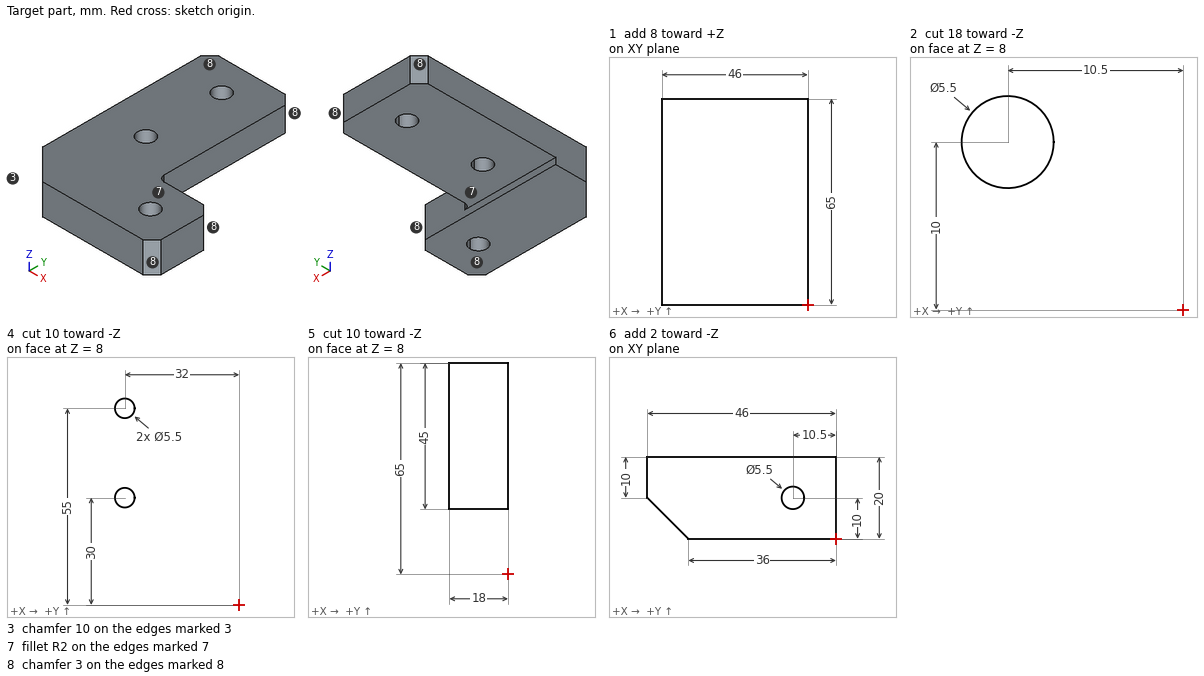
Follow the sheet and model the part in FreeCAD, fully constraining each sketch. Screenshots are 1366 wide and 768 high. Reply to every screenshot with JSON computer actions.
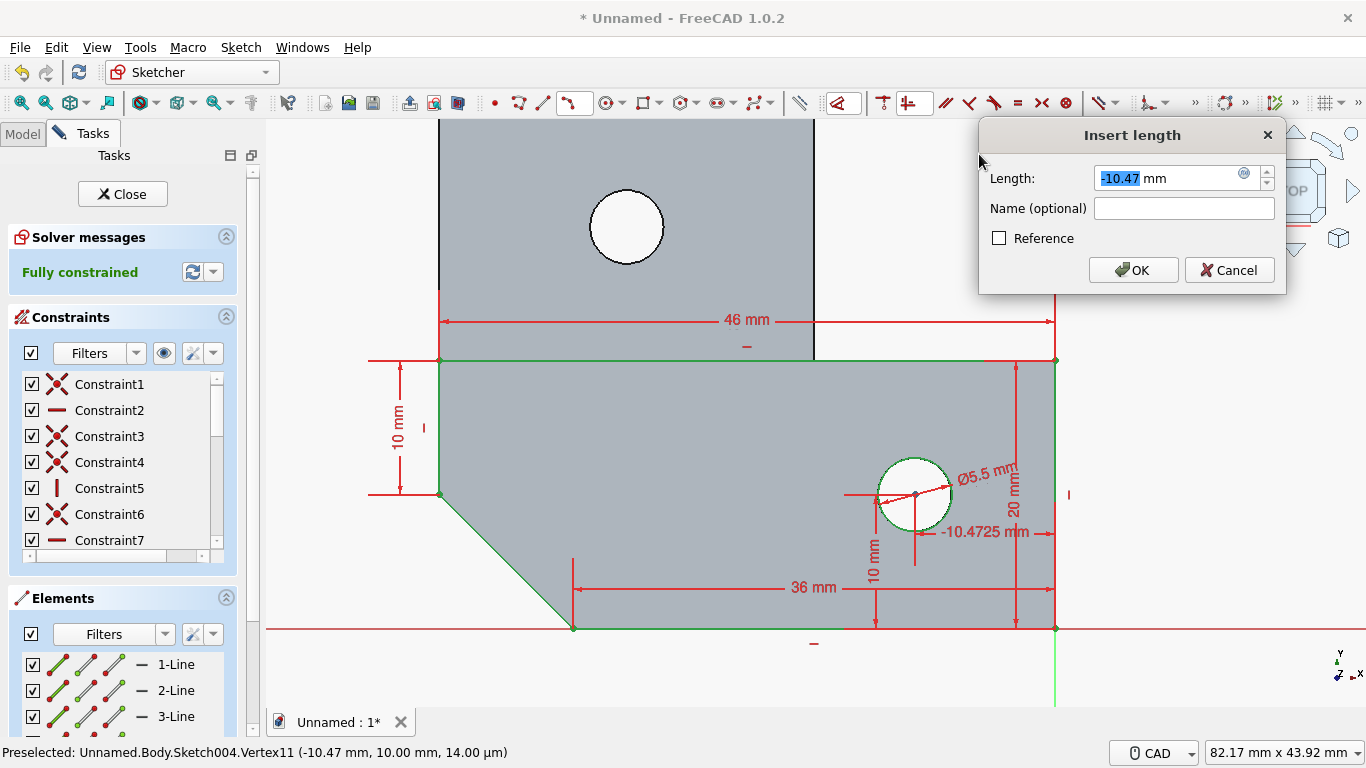
{"action": "type", "text": "-10.5"}
{"action": "key", "text": "Return"}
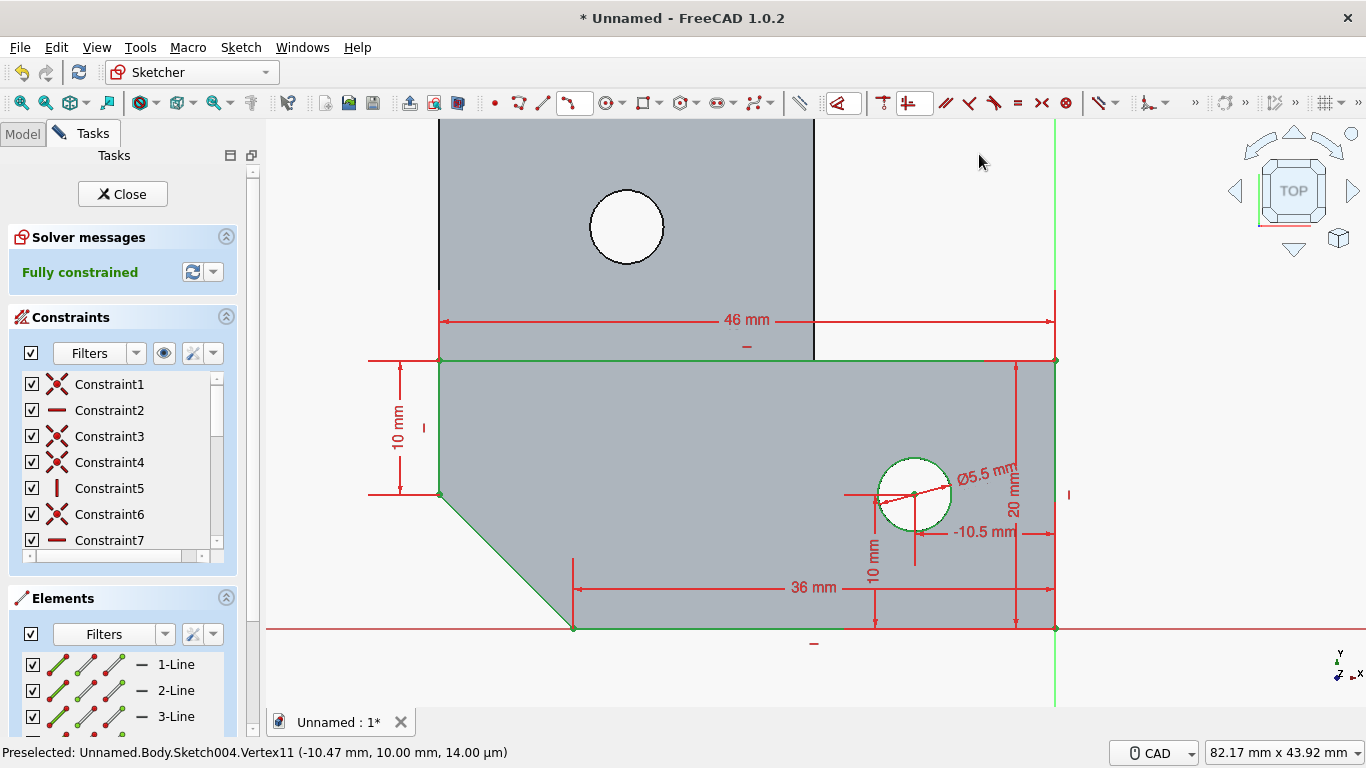
{"action": "left_click", "coordinate": [123, 194]}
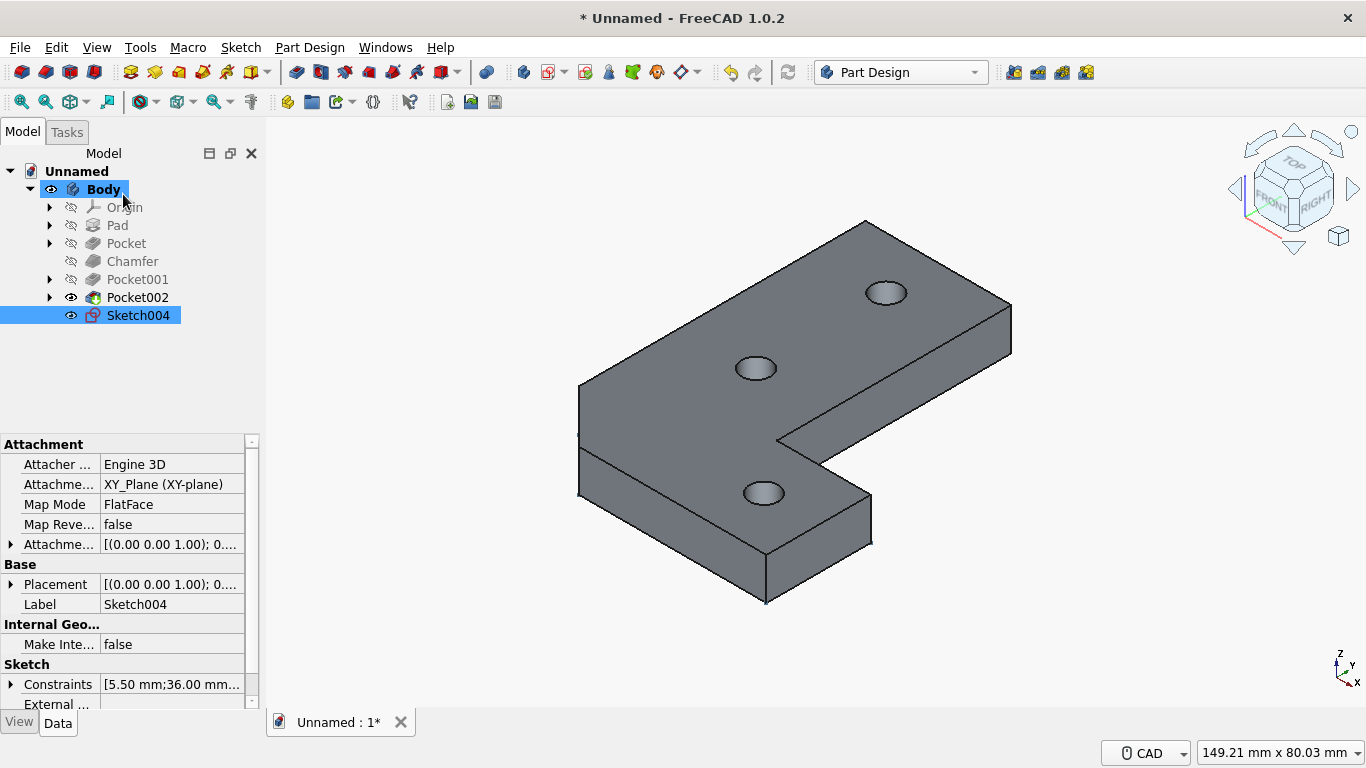
{"action": "left_click", "coordinate": [132, 72]}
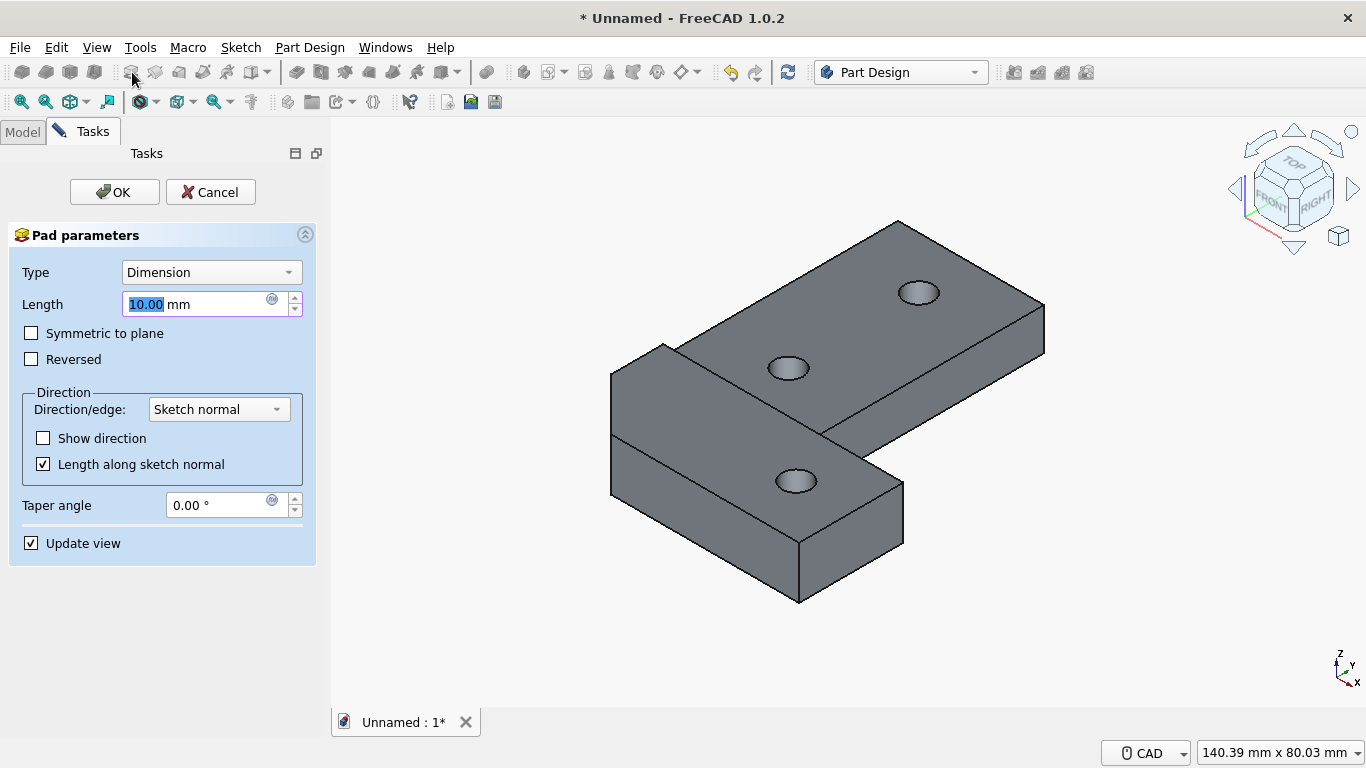
{"action": "type", "text": "2"}
{"action": "key", "text": "Tab"}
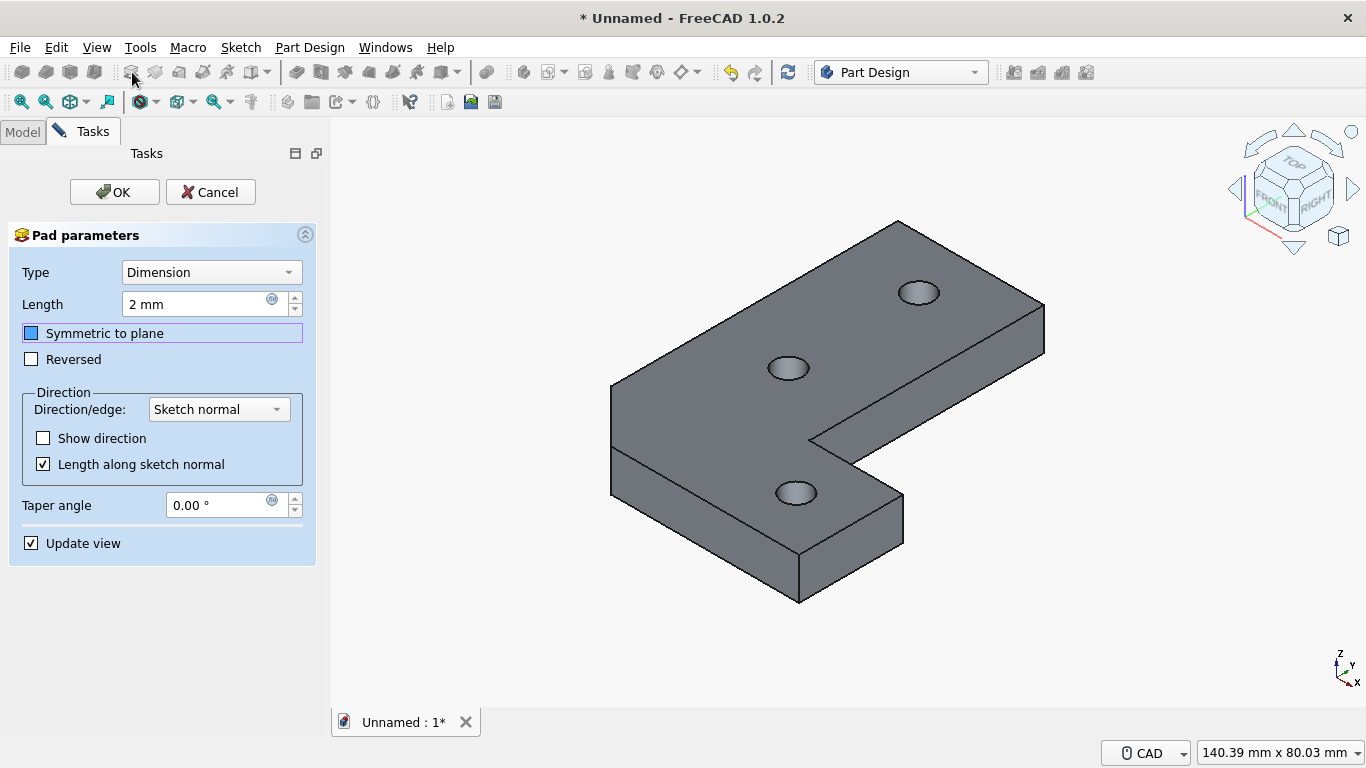
{"action": "left_click", "coordinate": [30, 359]}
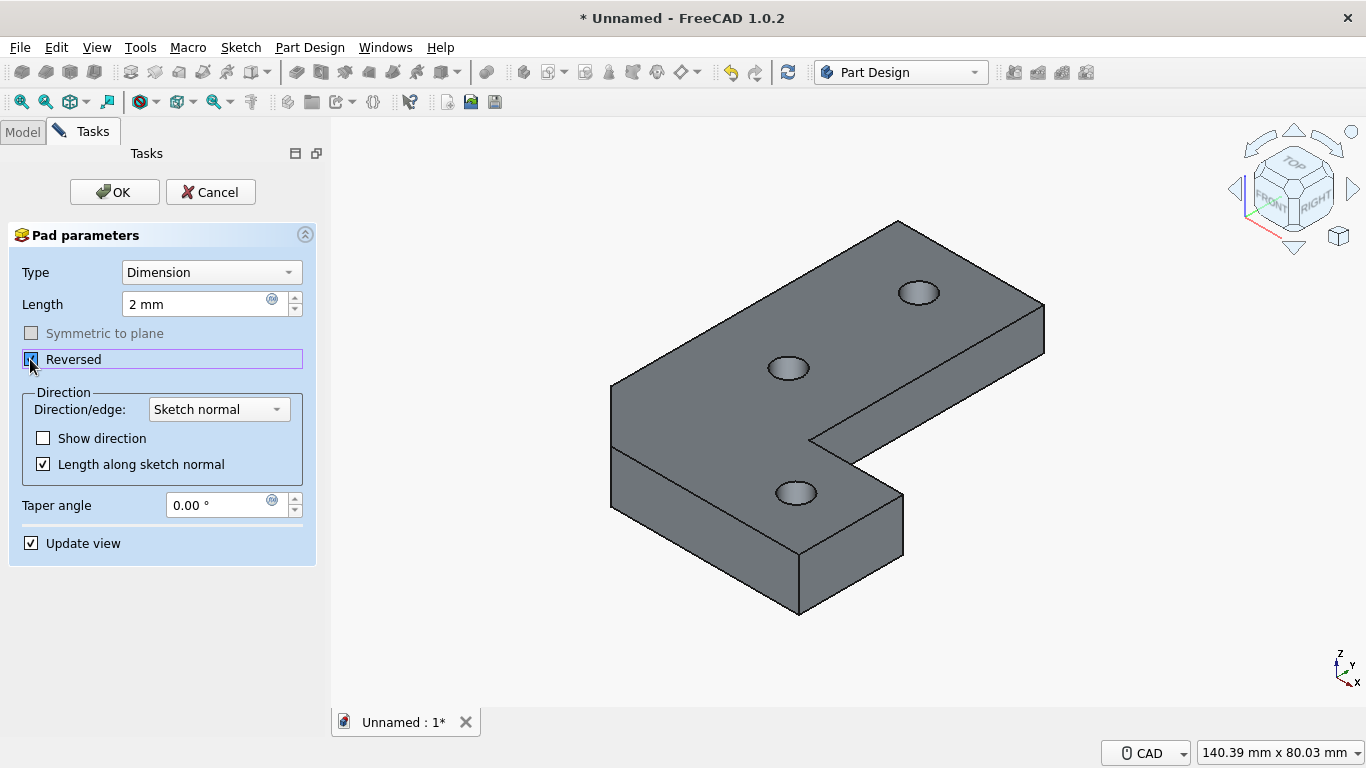
{"action": "left_click", "coordinate": [115, 192]}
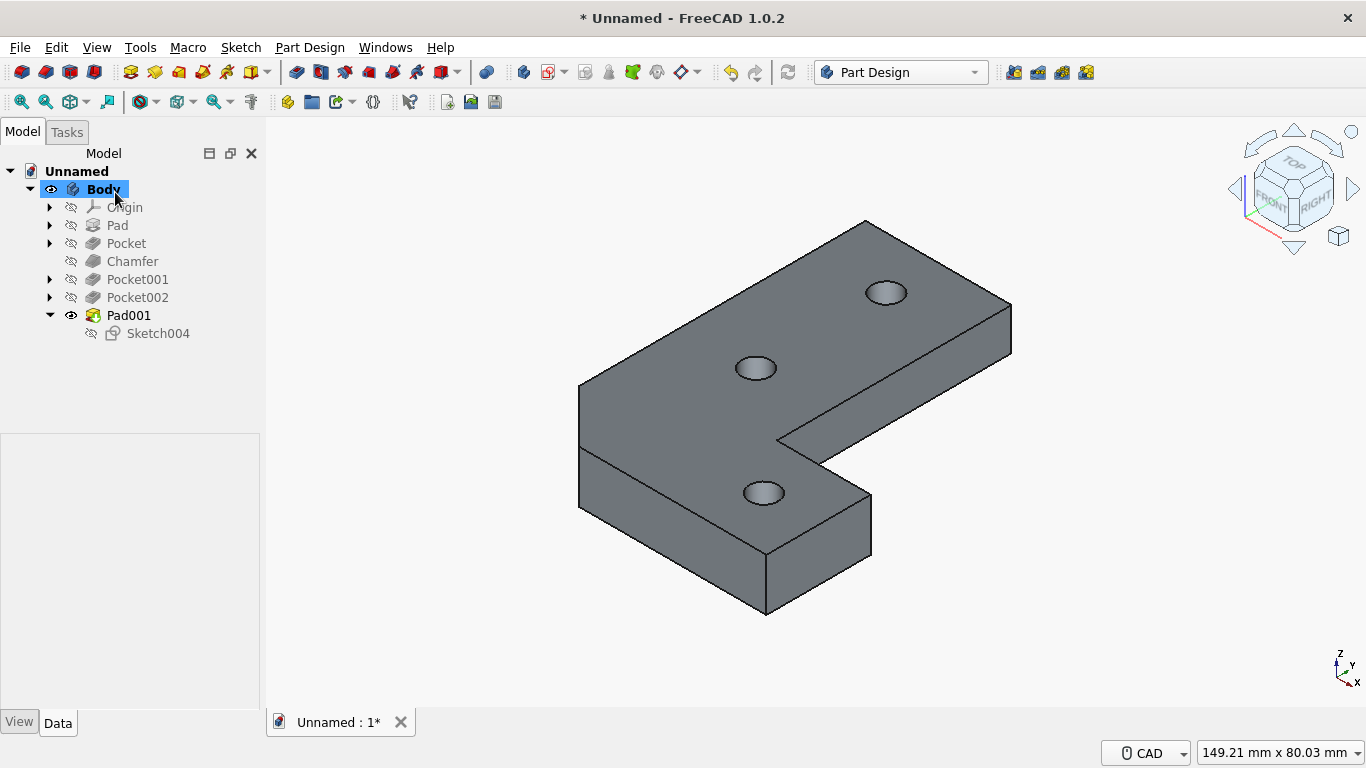
{"action": "key", "text": "2"}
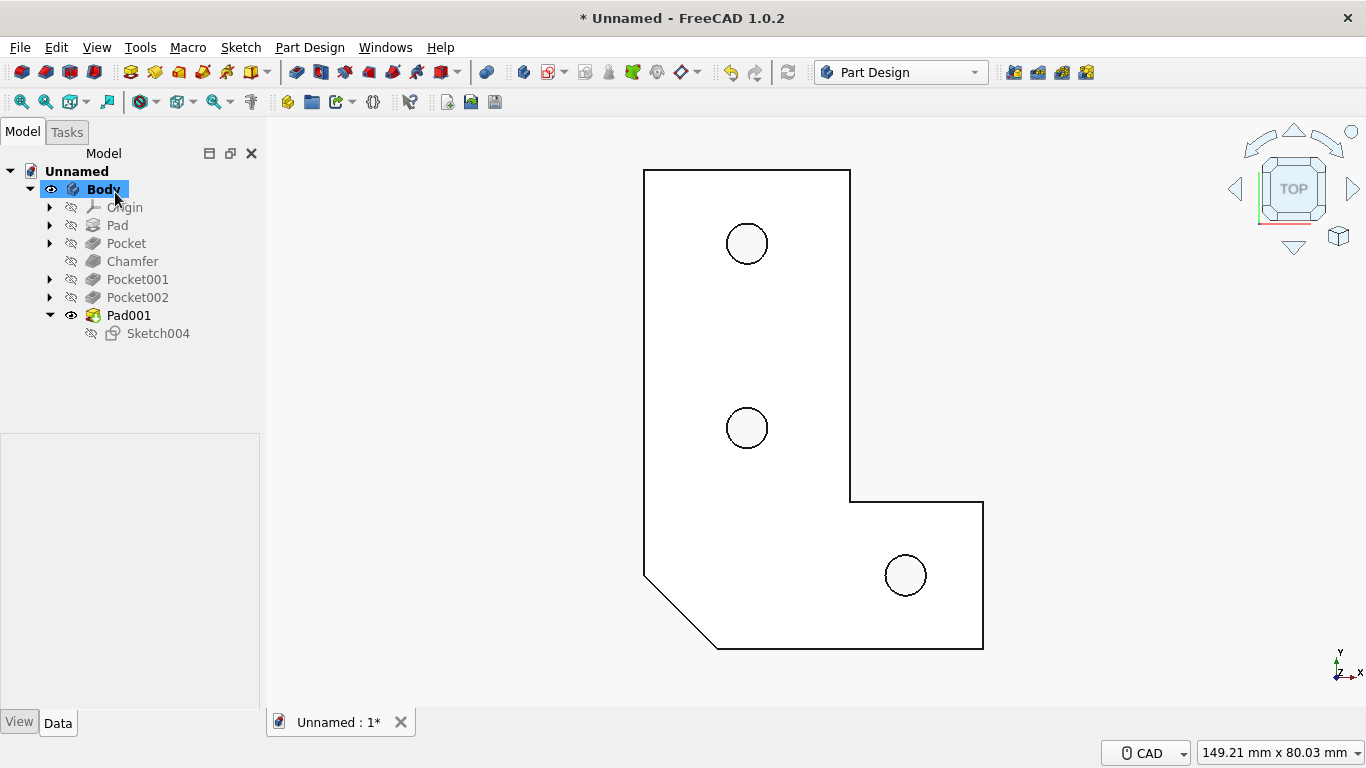
{"action": "key", "text": "0"}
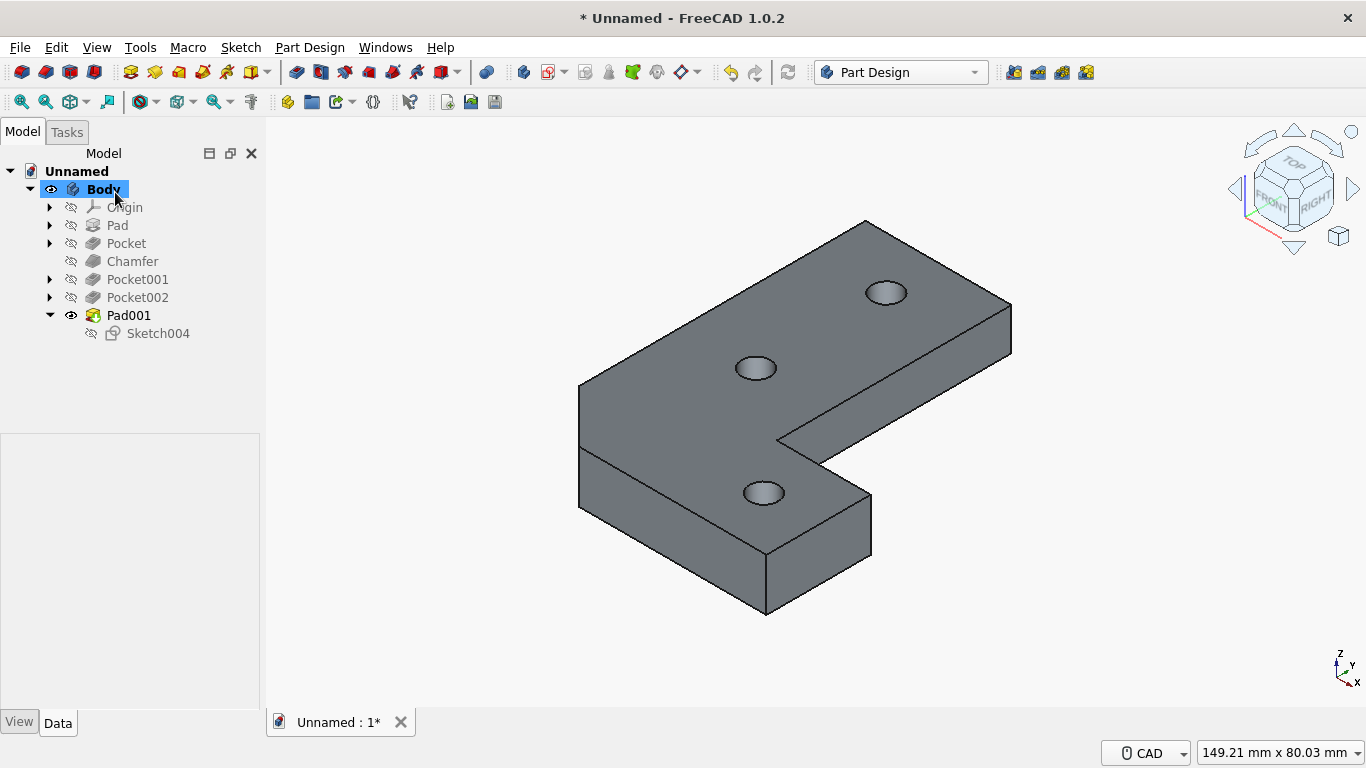
{"action": "key", "text": "1"}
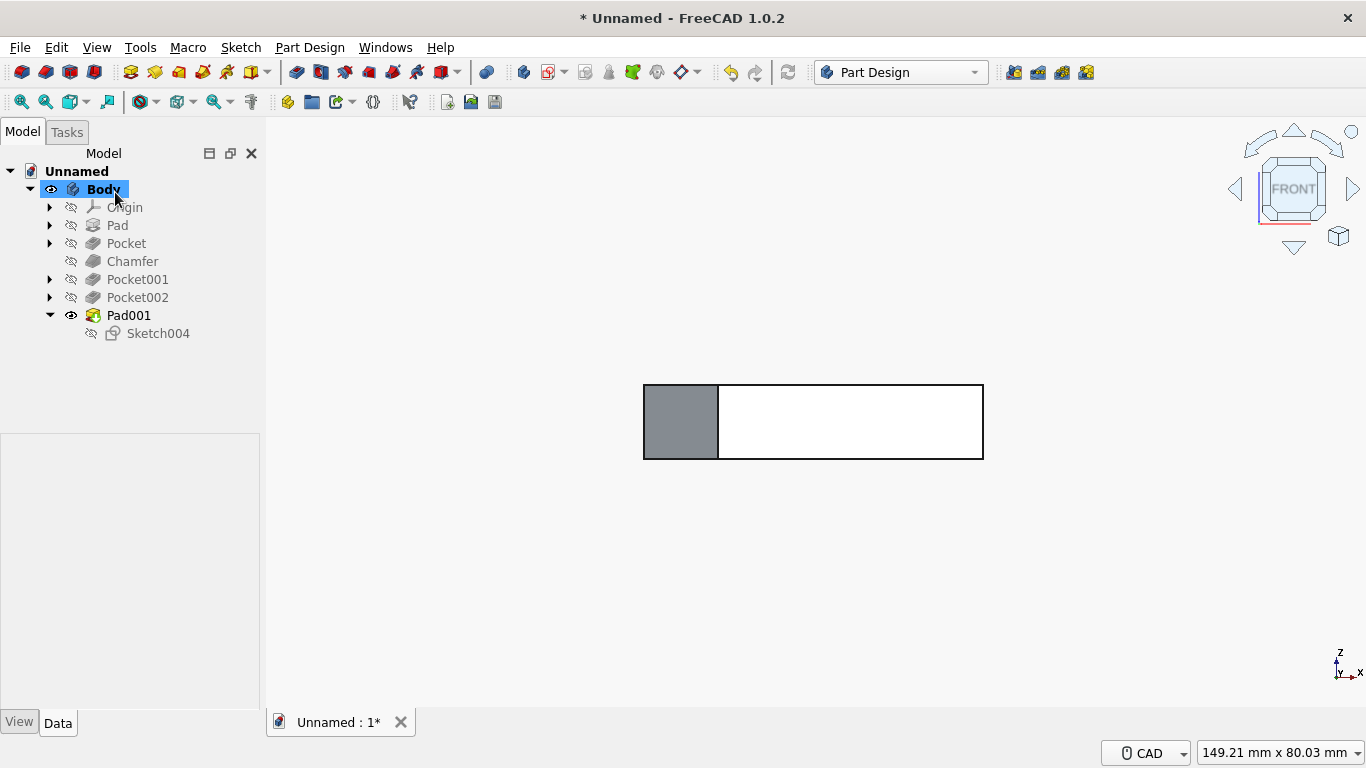
{"action": "key", "text": "v f"}